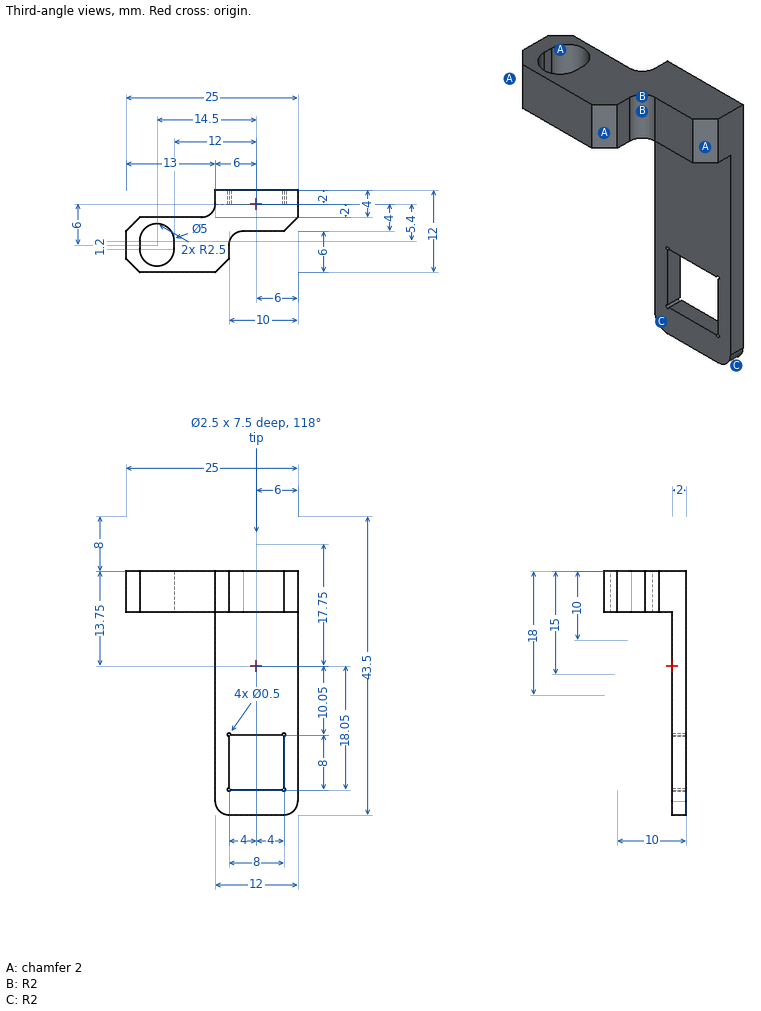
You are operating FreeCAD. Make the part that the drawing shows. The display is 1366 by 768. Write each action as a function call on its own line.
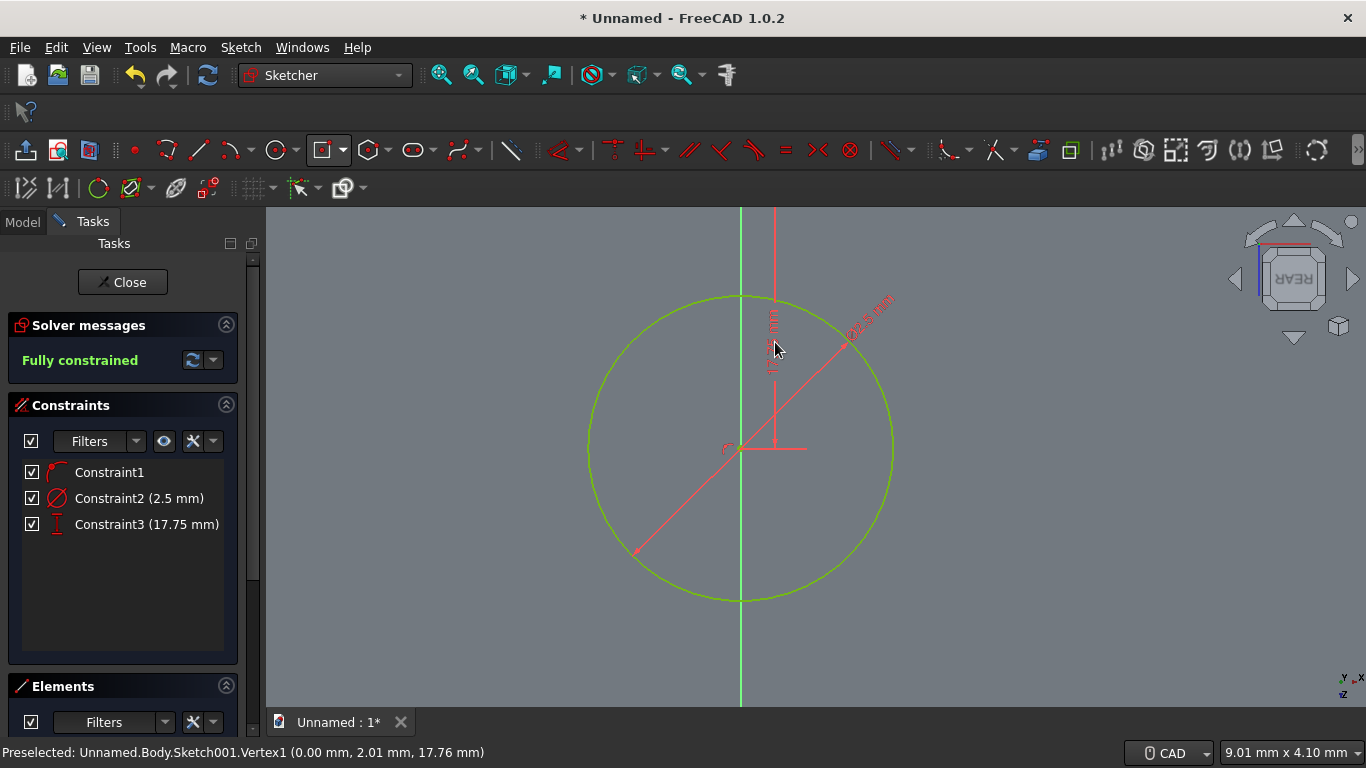
click(123, 282)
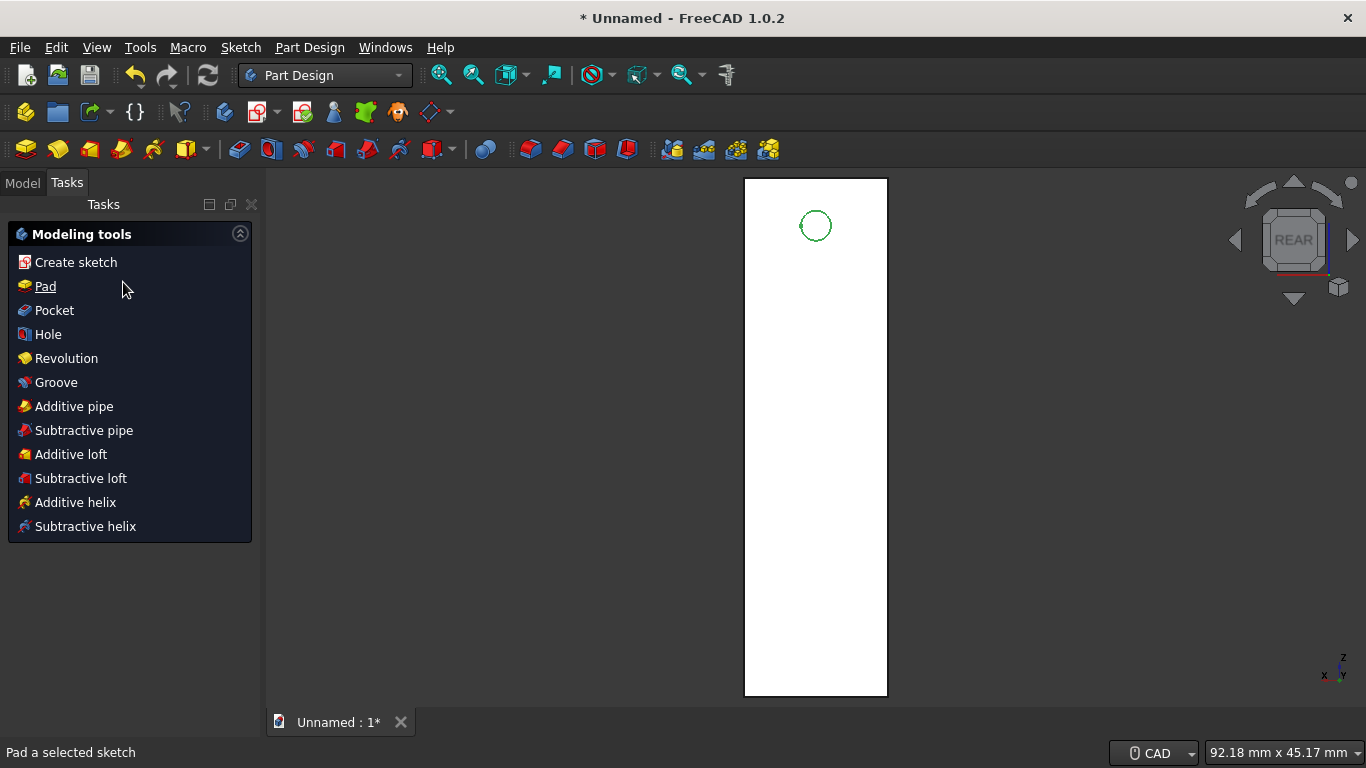
click(272, 150)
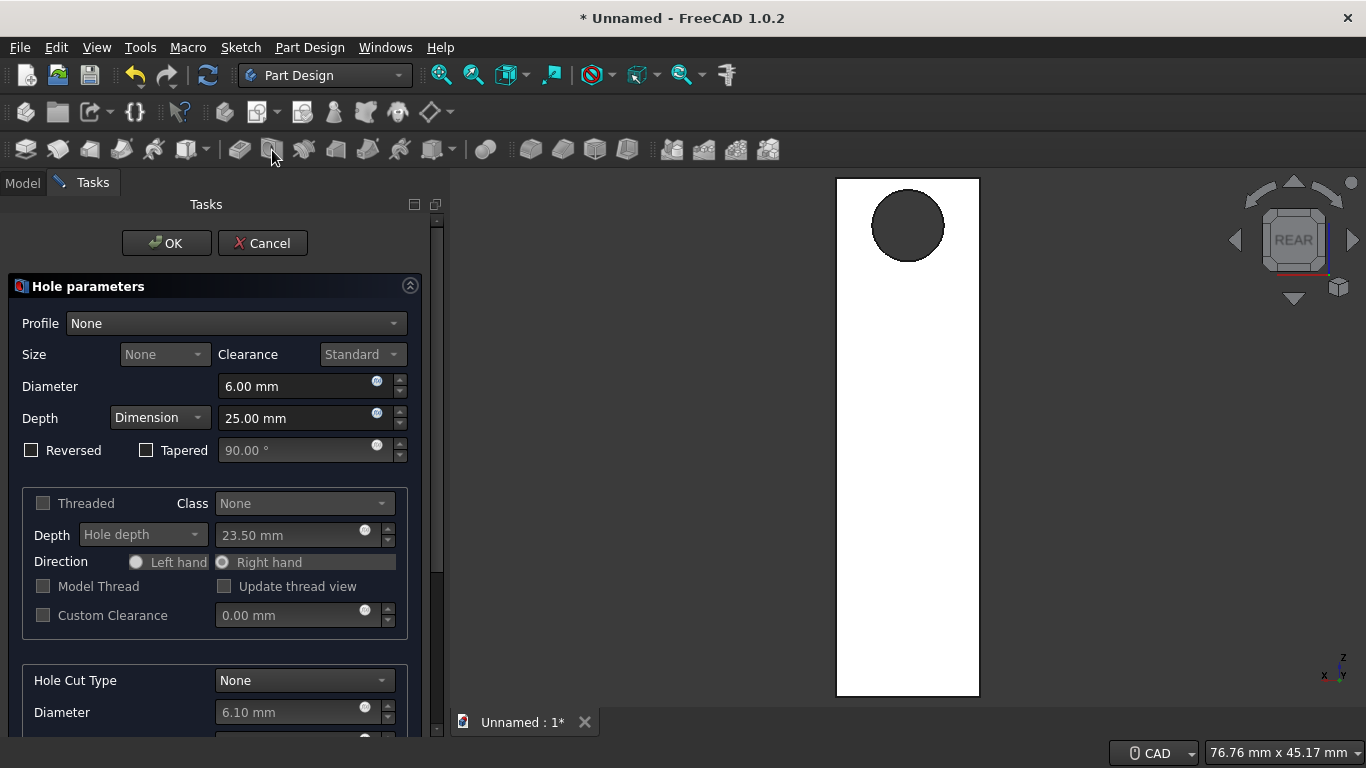
triple_click(305, 386)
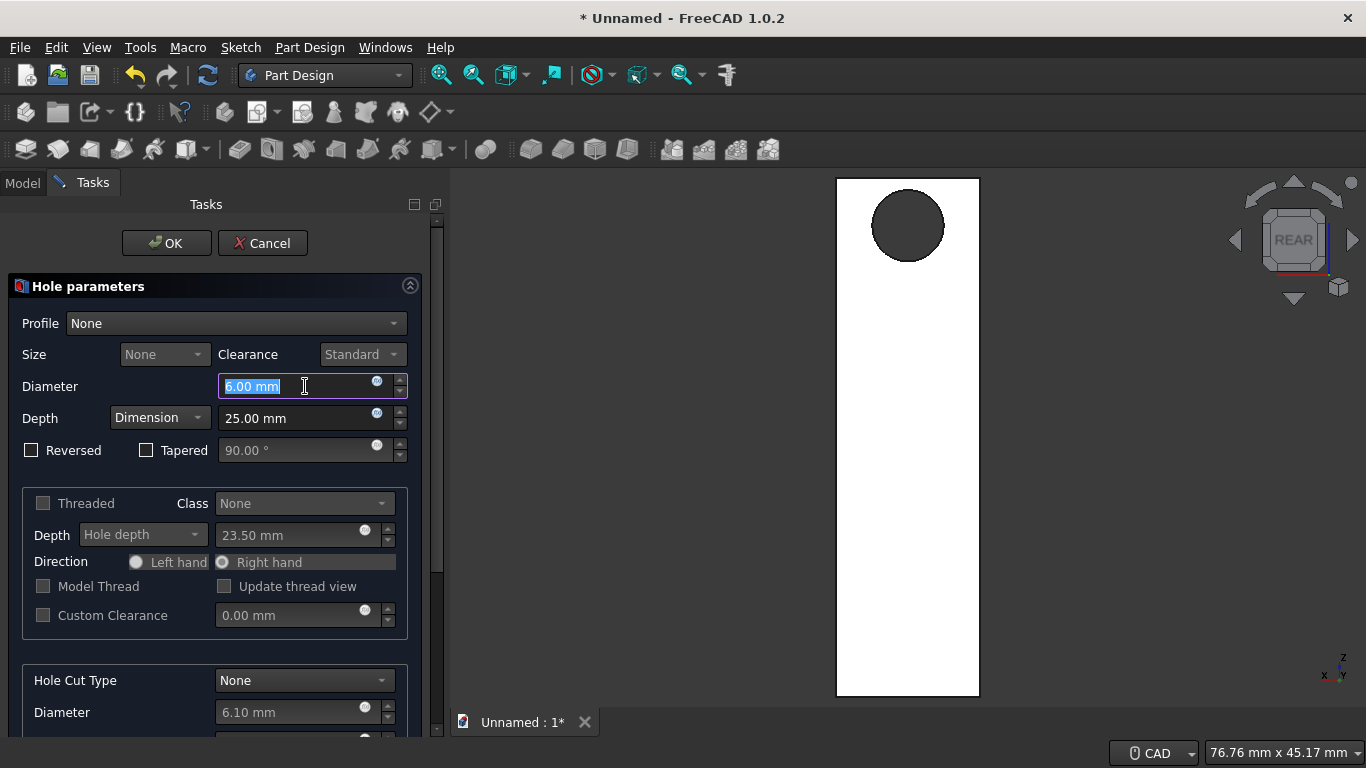
text(2.5)
key(Tab)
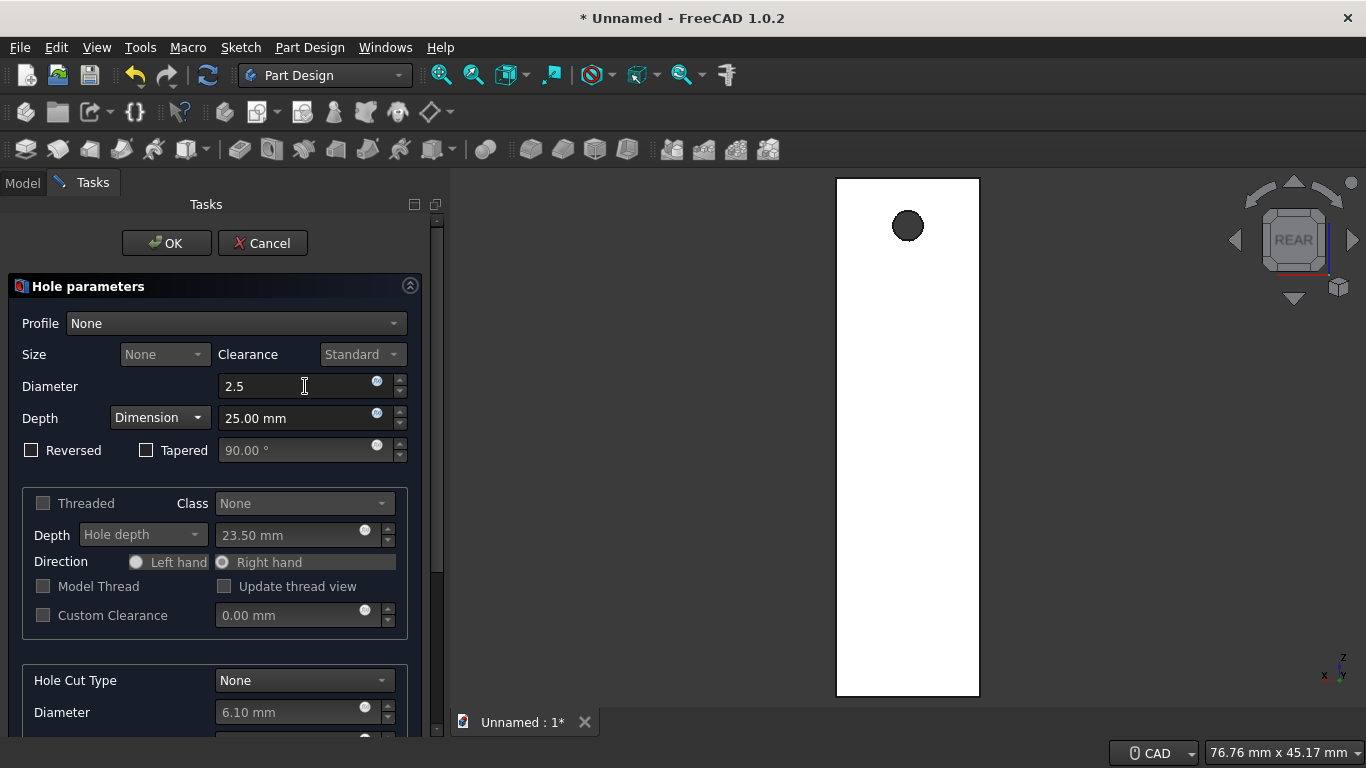
triple_click(305, 418)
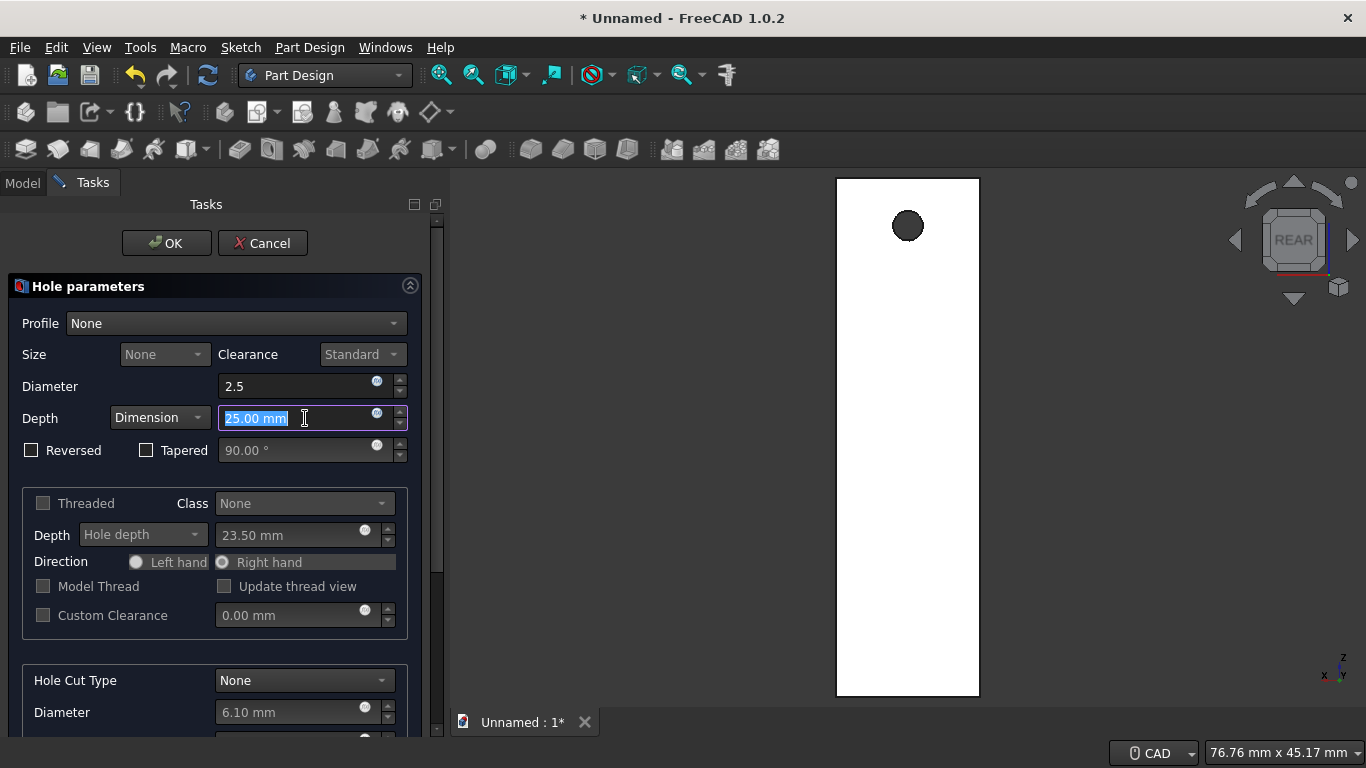
text(7.5)
key(Tab)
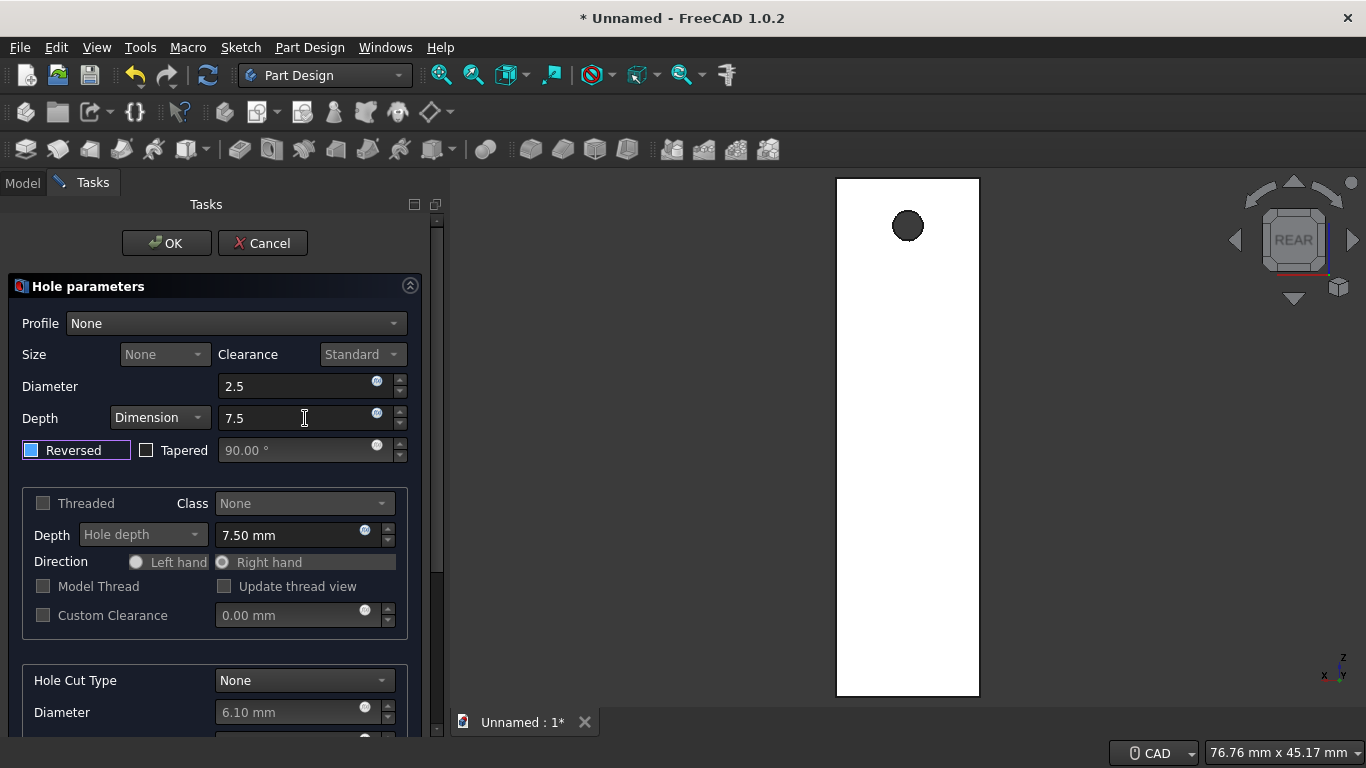
click(167, 243)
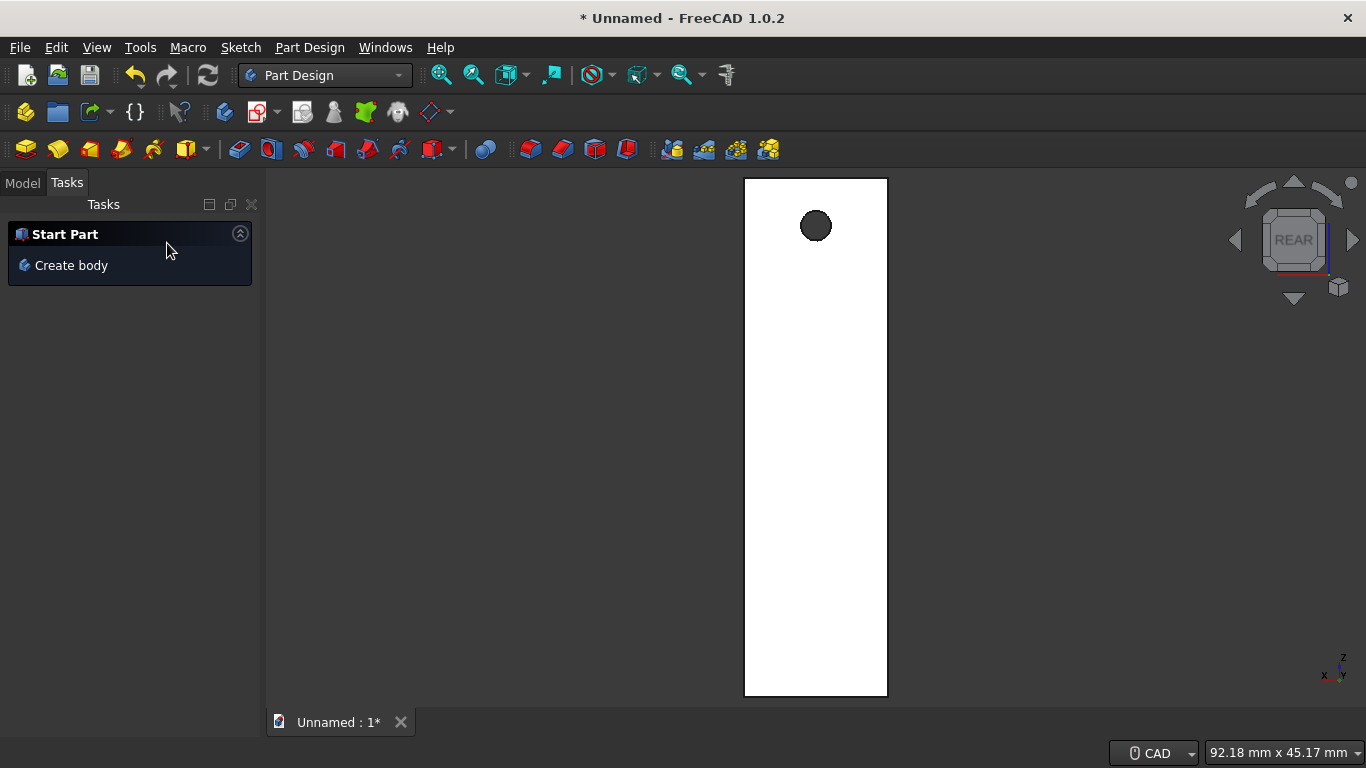
key(0)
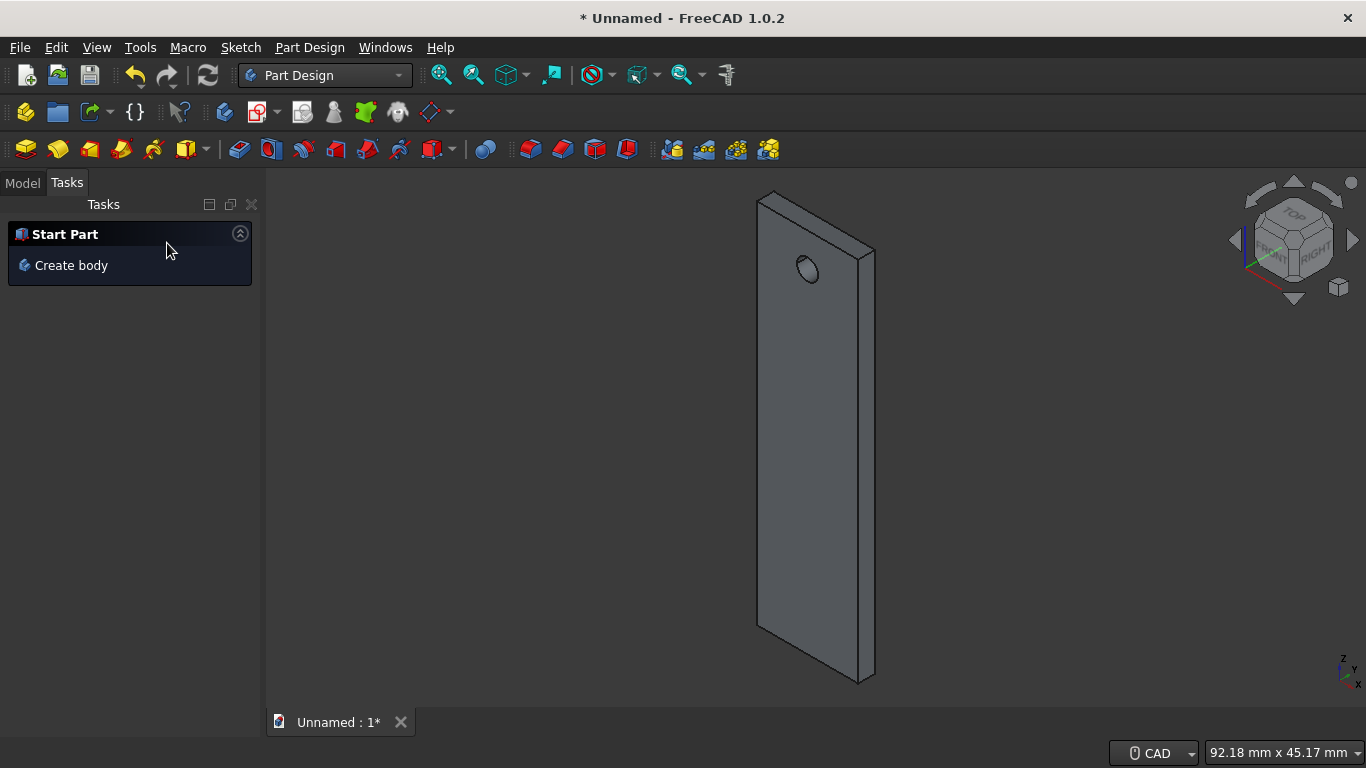
key(2)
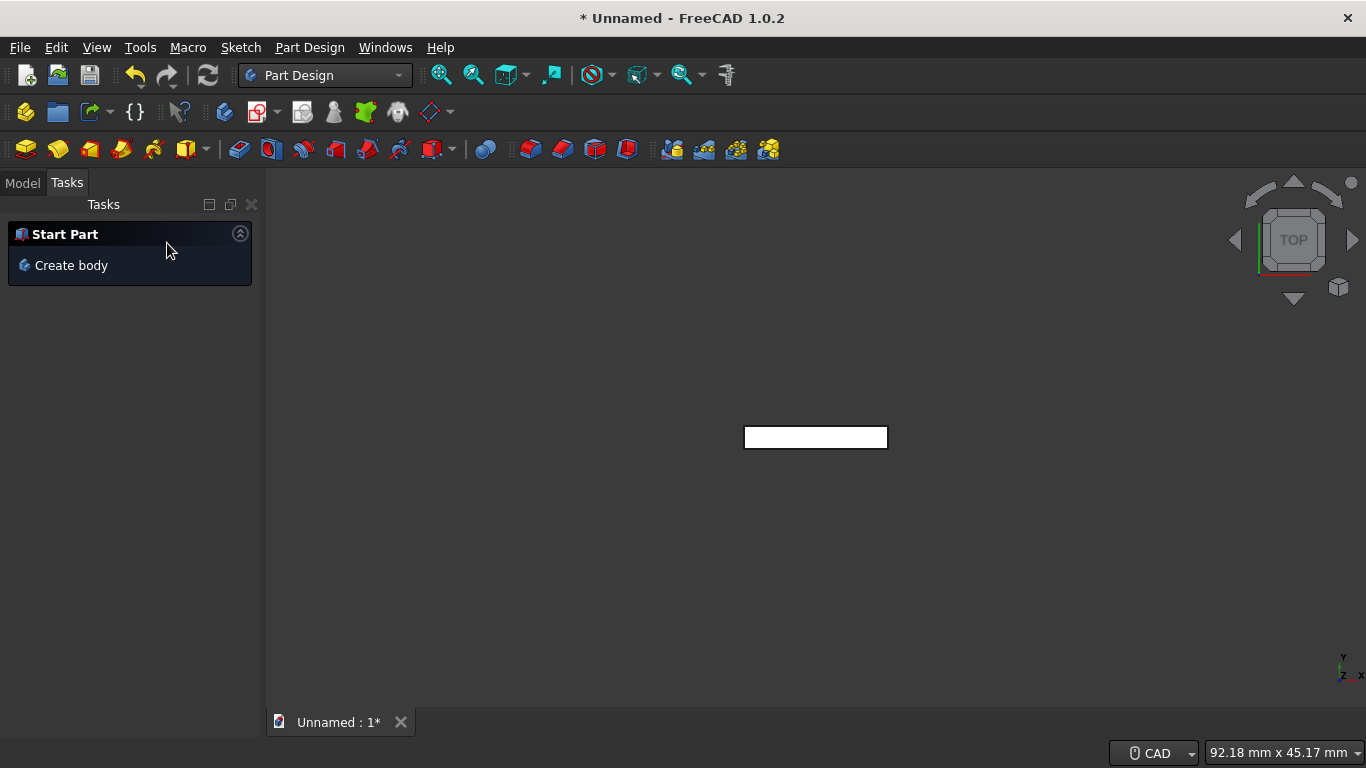
click(442, 76)